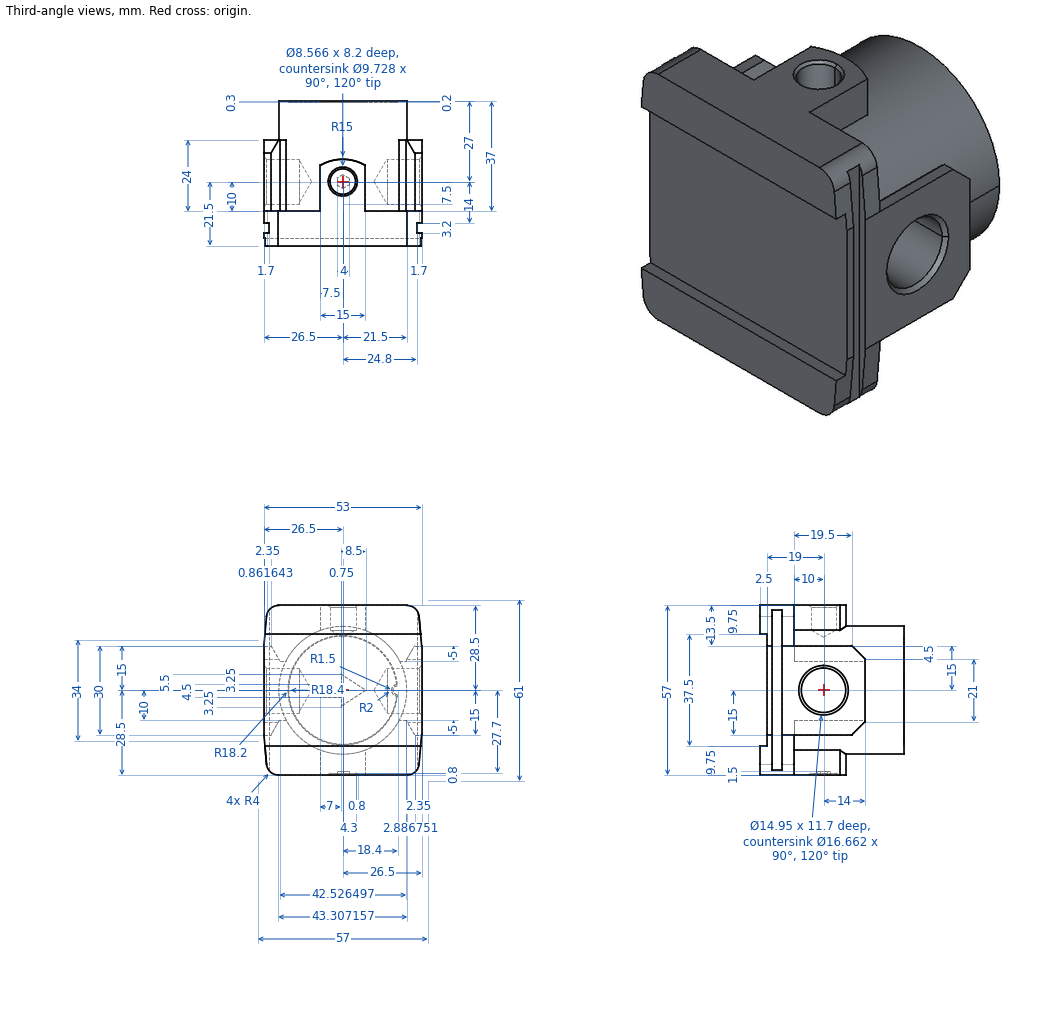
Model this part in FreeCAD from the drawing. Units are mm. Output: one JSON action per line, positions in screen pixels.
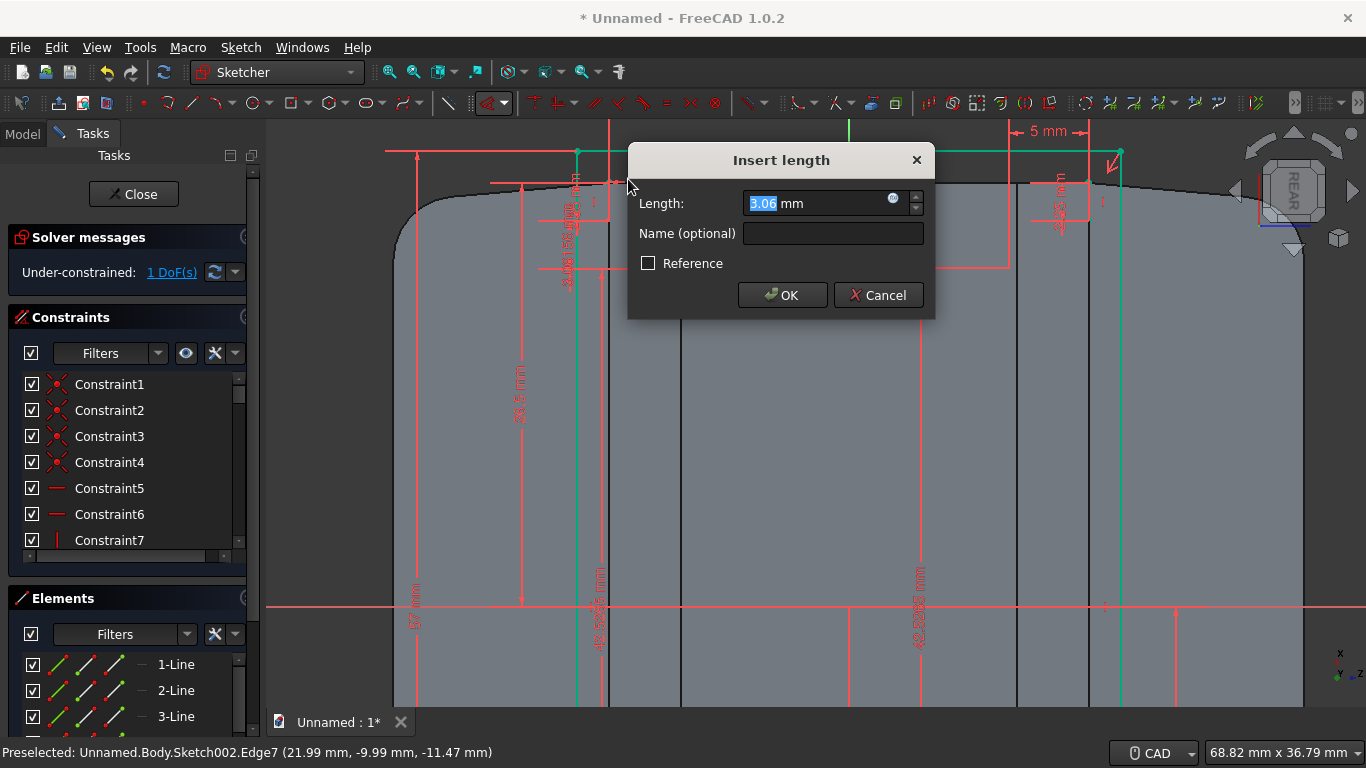
{"action": "type", "text": "2.886751"}
{"action": "key", "text": "Return"}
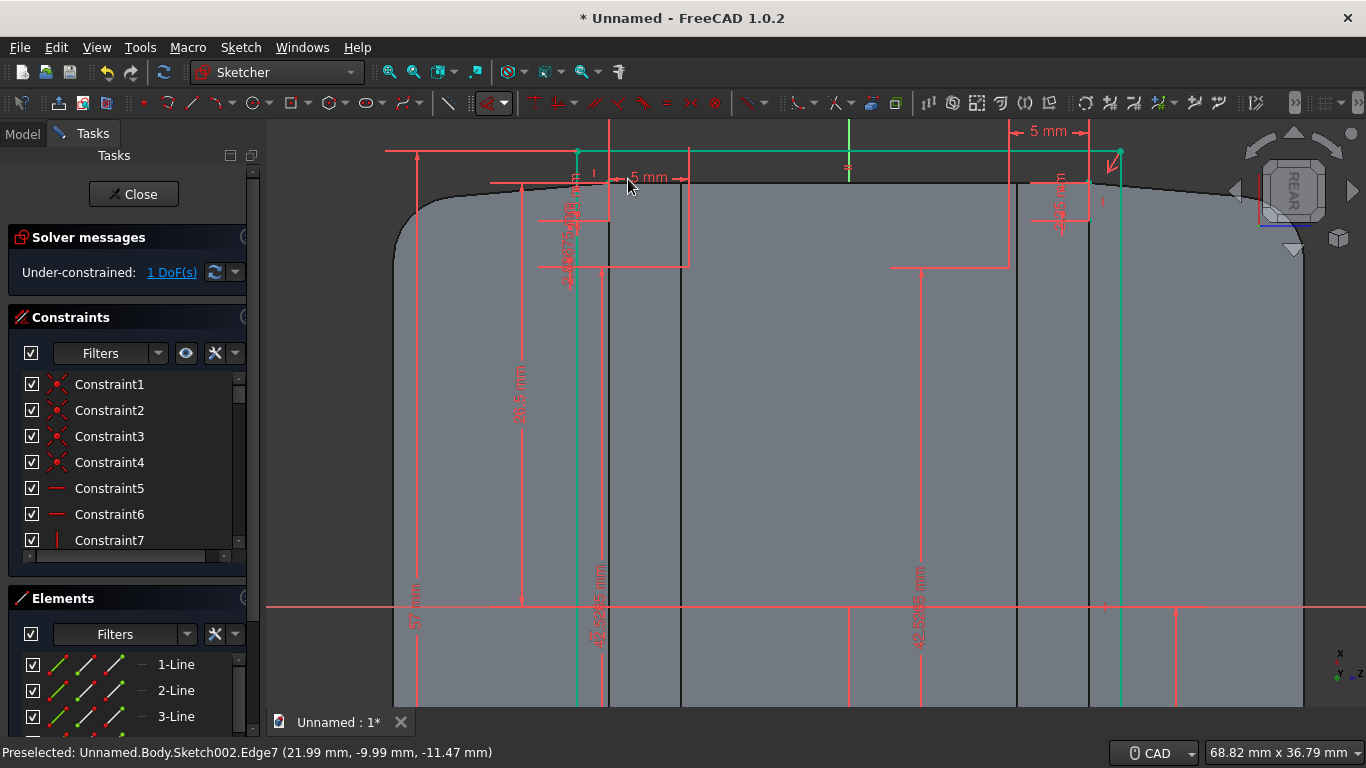
{"action": "left_click", "coordinate": [1065, 235]}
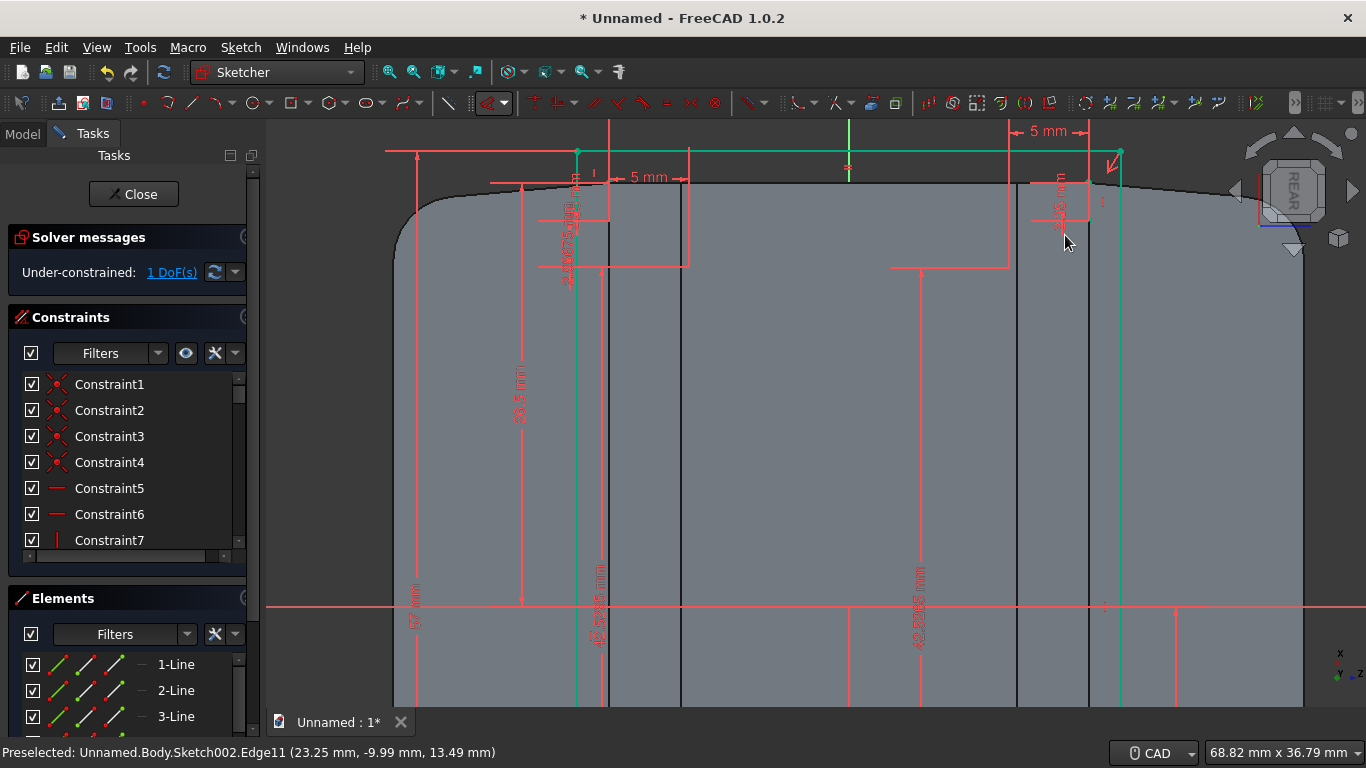
{"action": "key", "text": "i"}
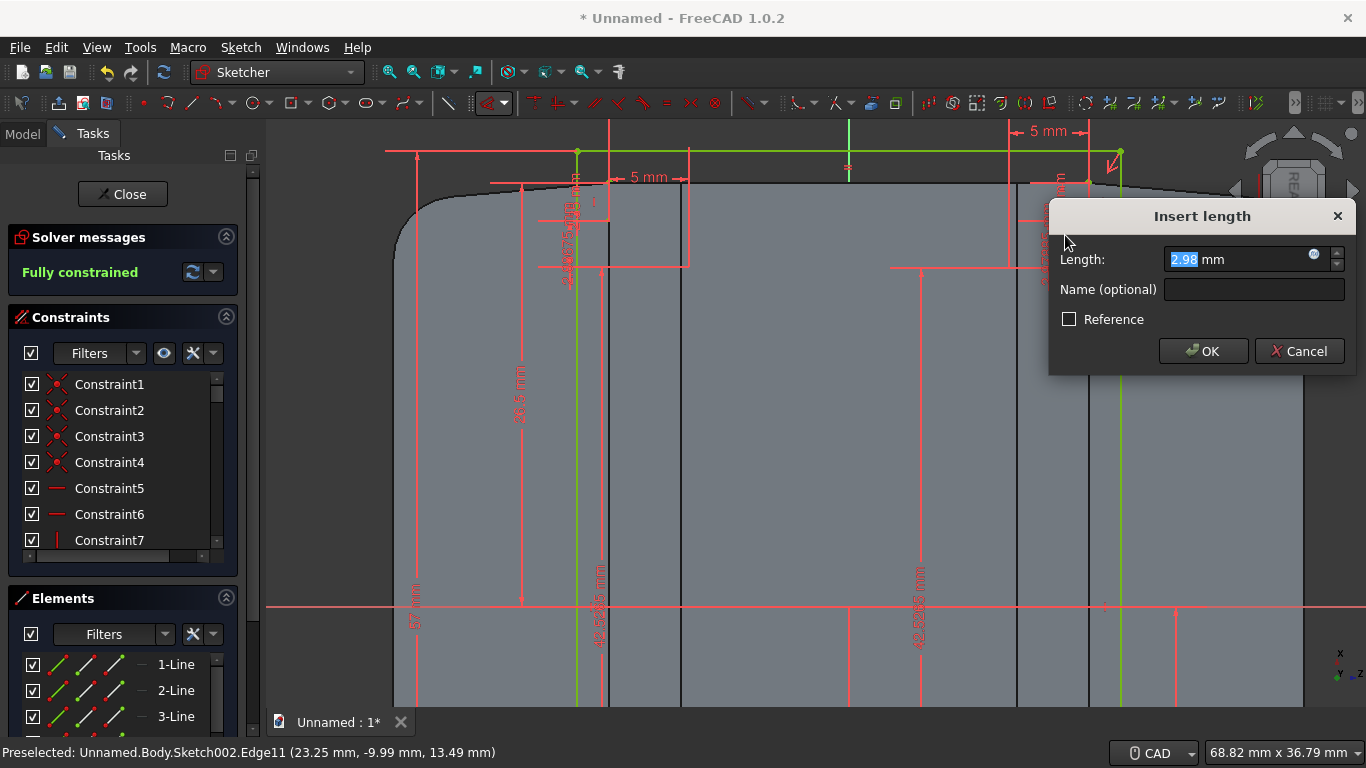
{"action": "type", "text": "2.886751"}
{"action": "key", "text": "Return"}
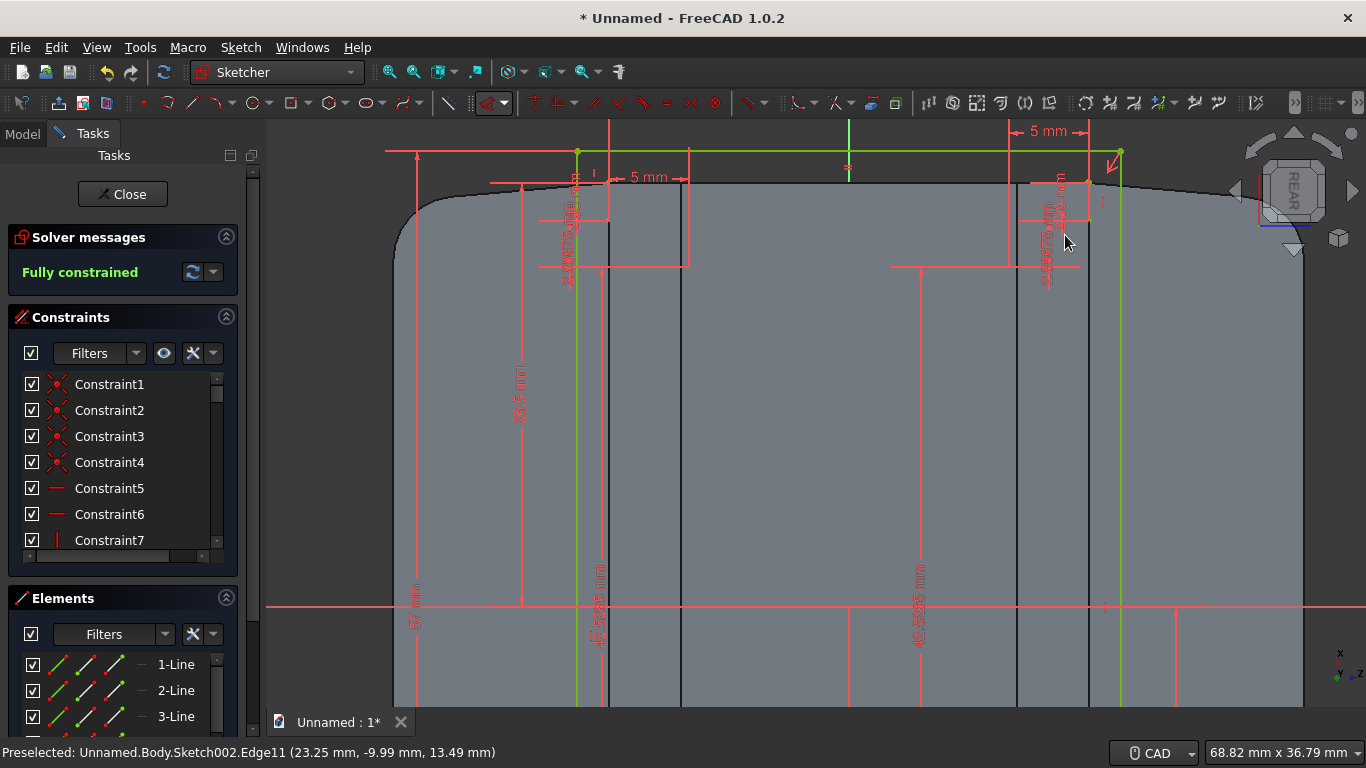
{"action": "left_click", "coordinate": [123, 194]}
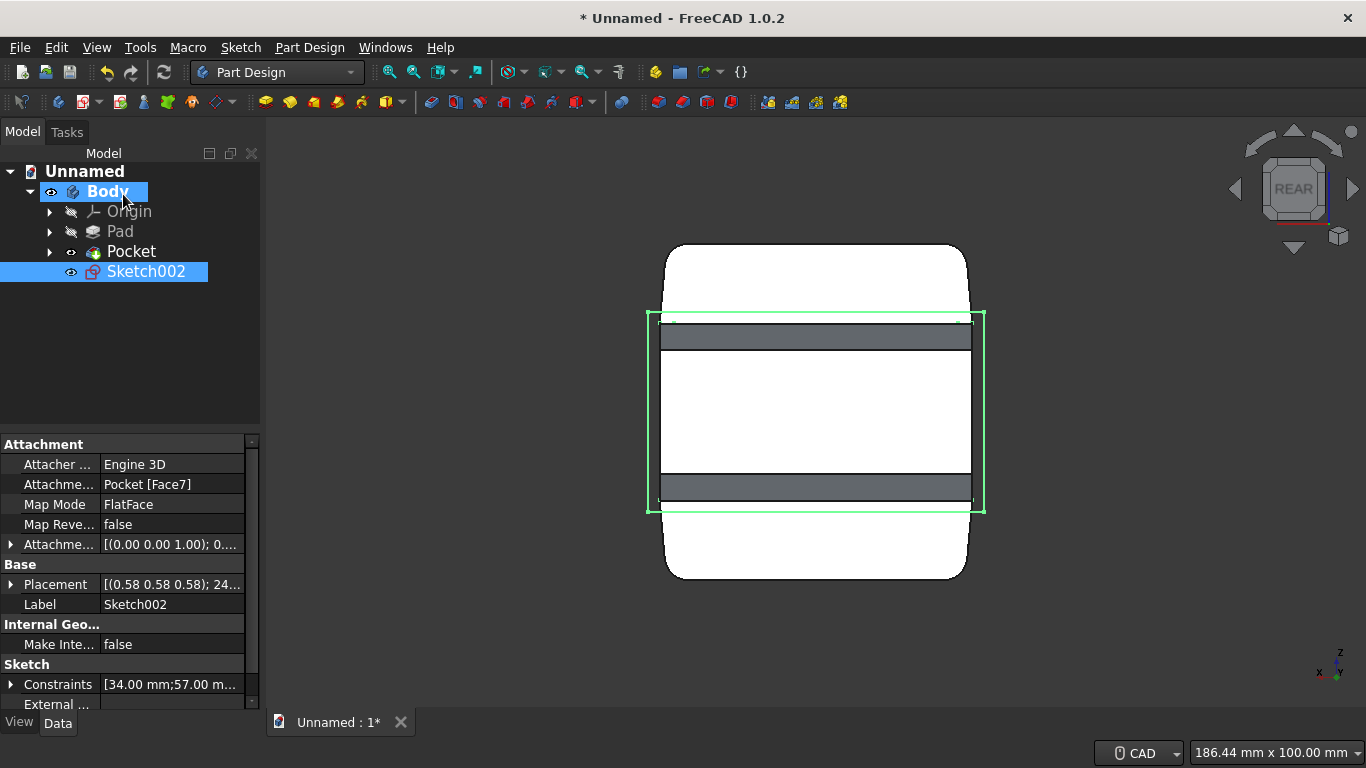
{"action": "left_click", "coordinate": [432, 102]}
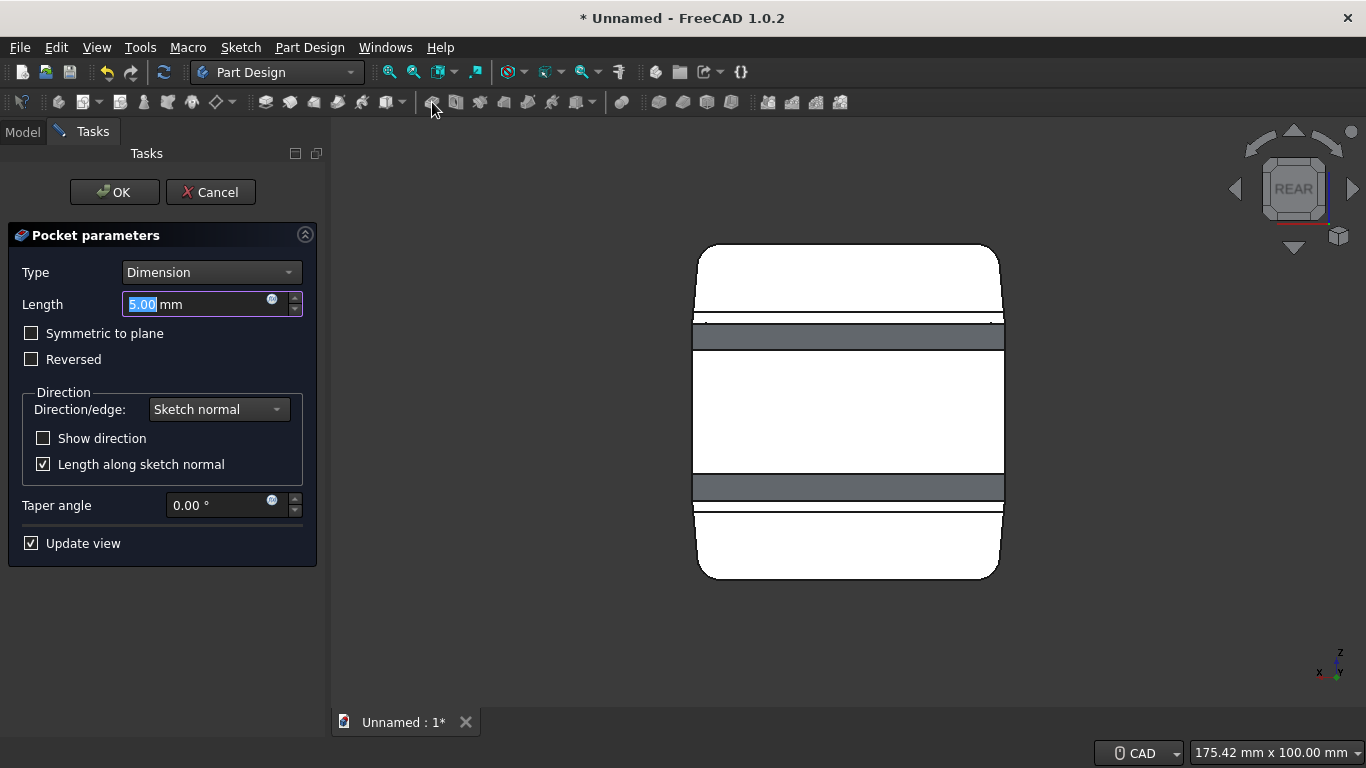
{"action": "type", "text": "24"}
{"action": "key", "text": "Tab"}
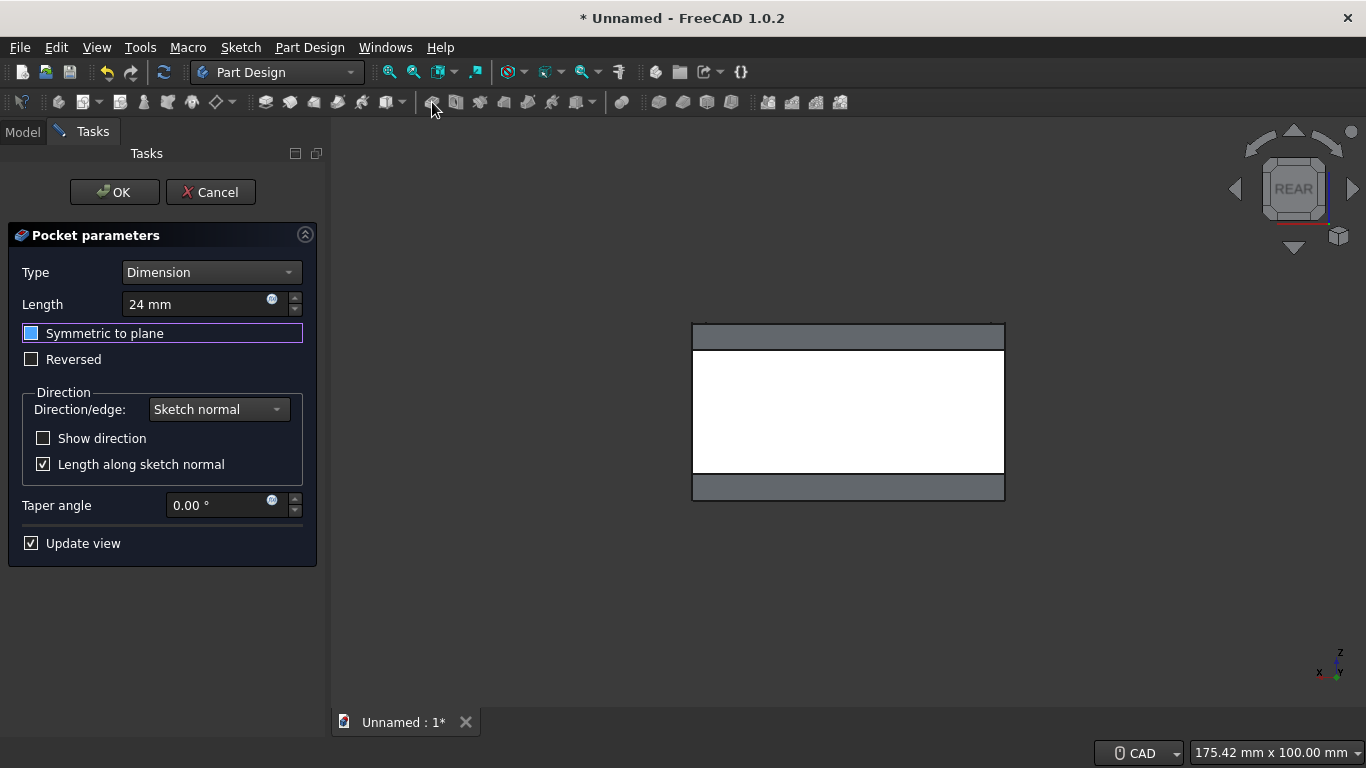
{"action": "left_click", "coordinate": [30, 359]}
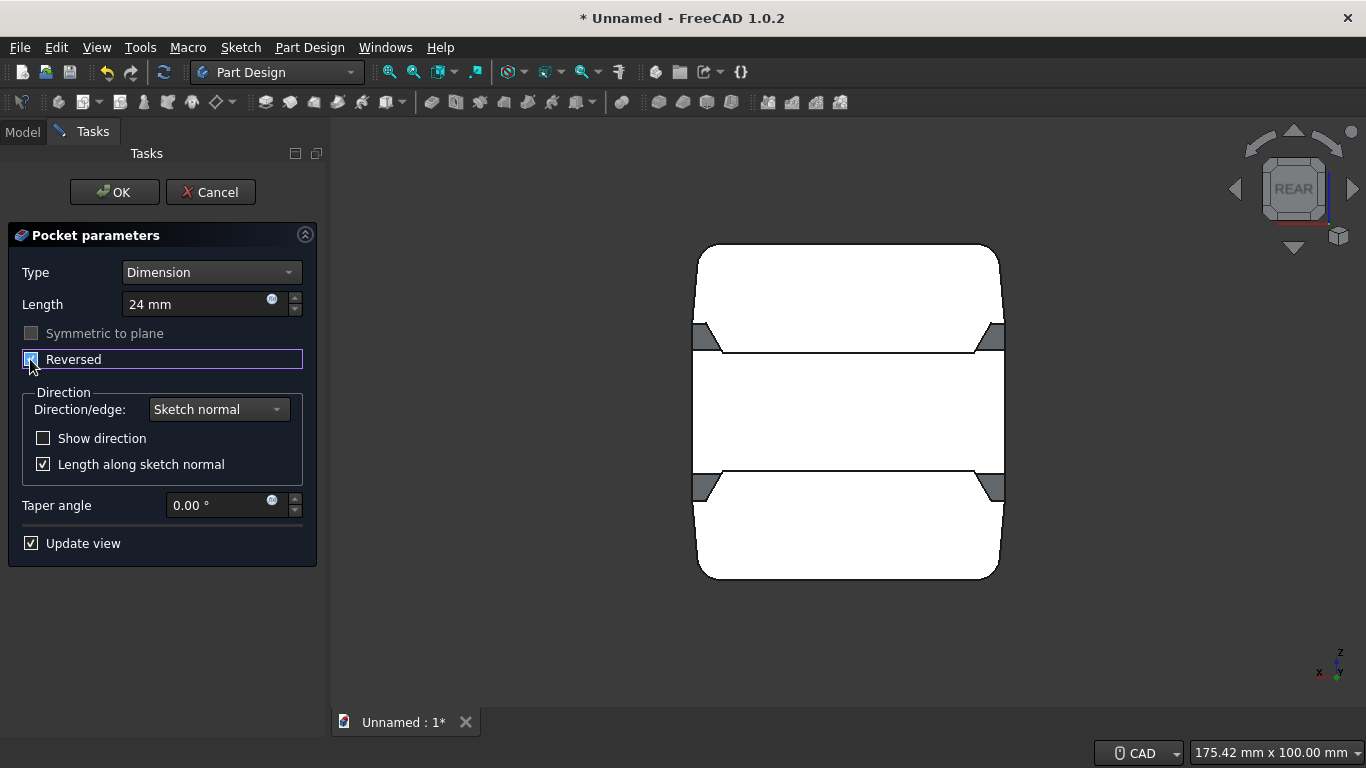
{"action": "left_click", "coordinate": [115, 192]}